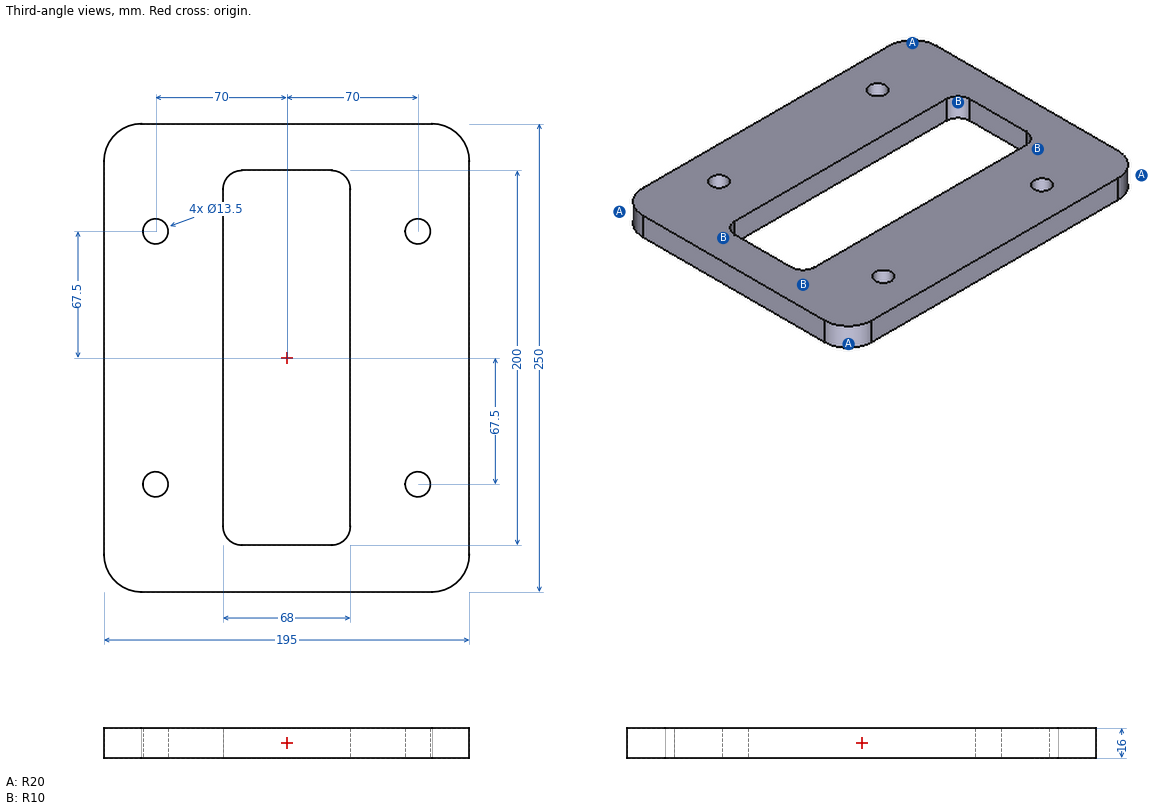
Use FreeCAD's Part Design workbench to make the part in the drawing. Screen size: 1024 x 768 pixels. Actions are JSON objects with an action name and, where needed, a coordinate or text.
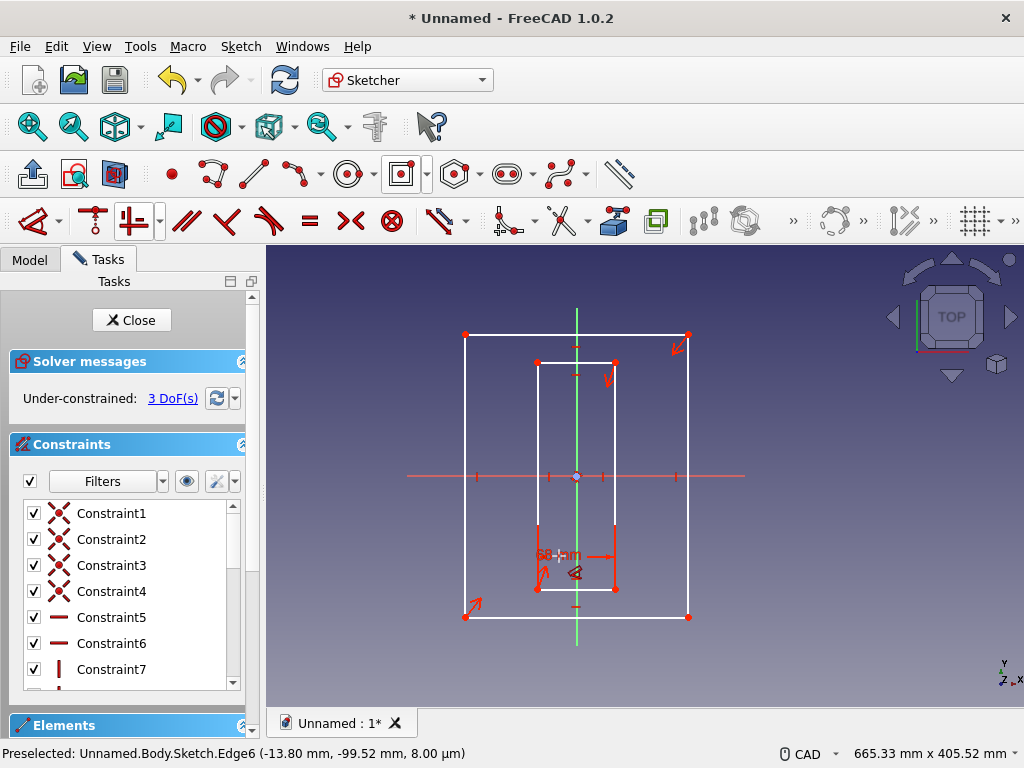
{"action": "left_click", "coordinate": [532, 618]}
{"action": "left_click", "coordinate": [526, 652]}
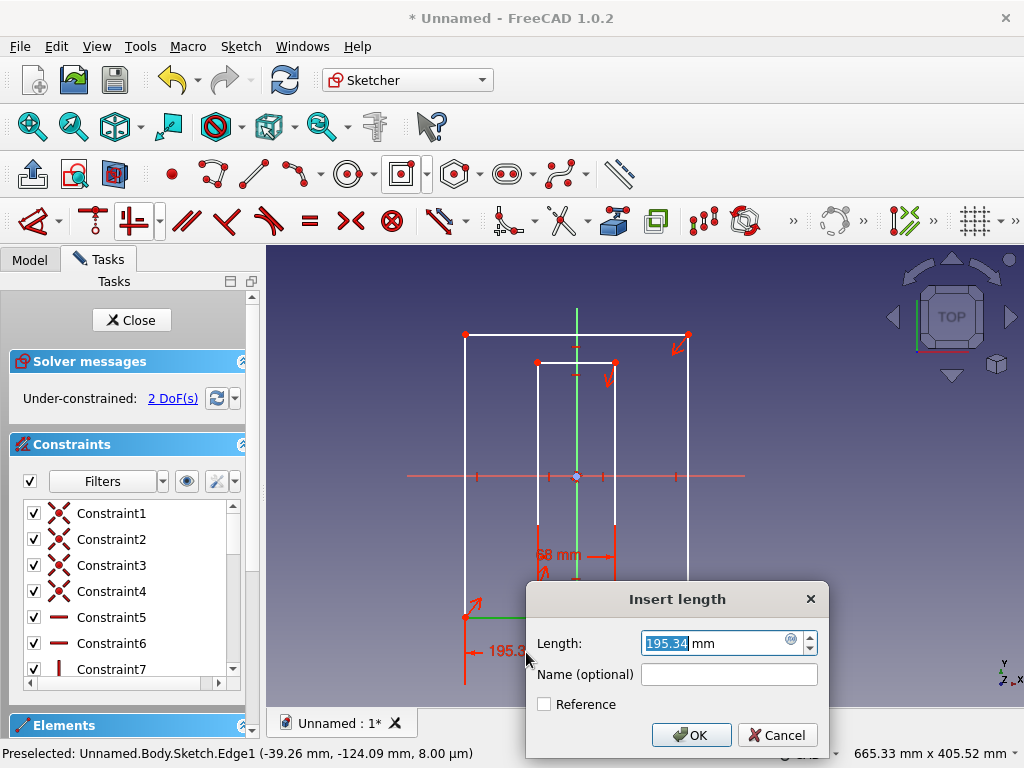
{"action": "type", "text": "195"}
{"action": "key", "text": "Return"}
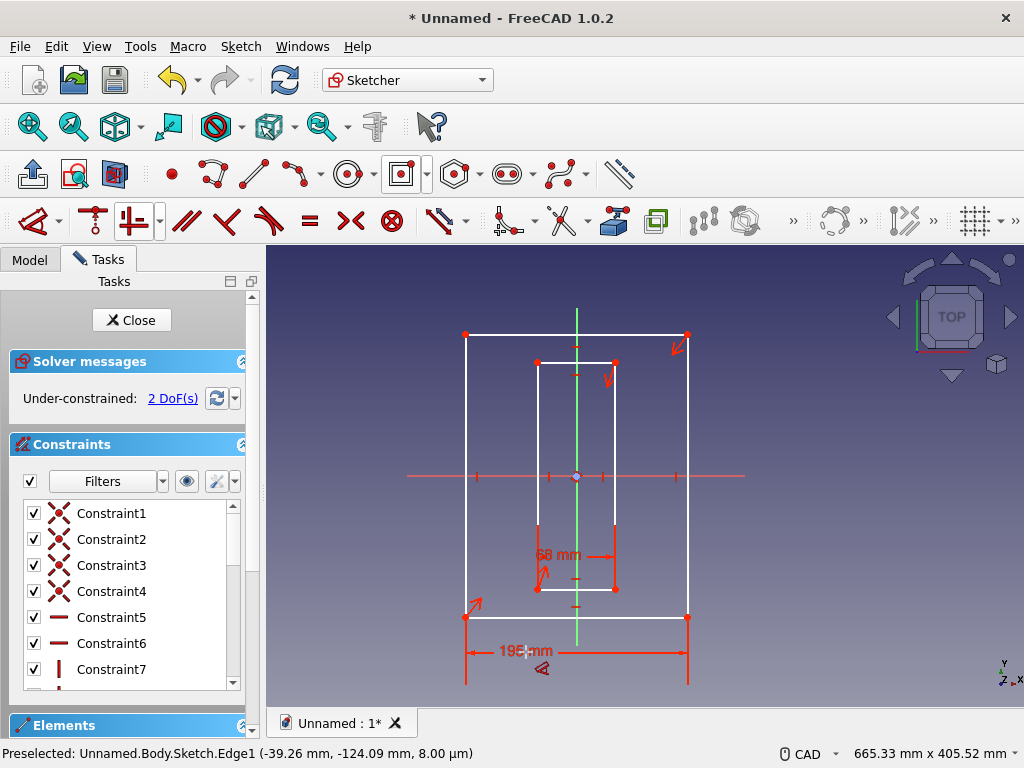
{"action": "left_click", "coordinate": [688, 533]}
{"action": "left_click", "coordinate": [722, 411]}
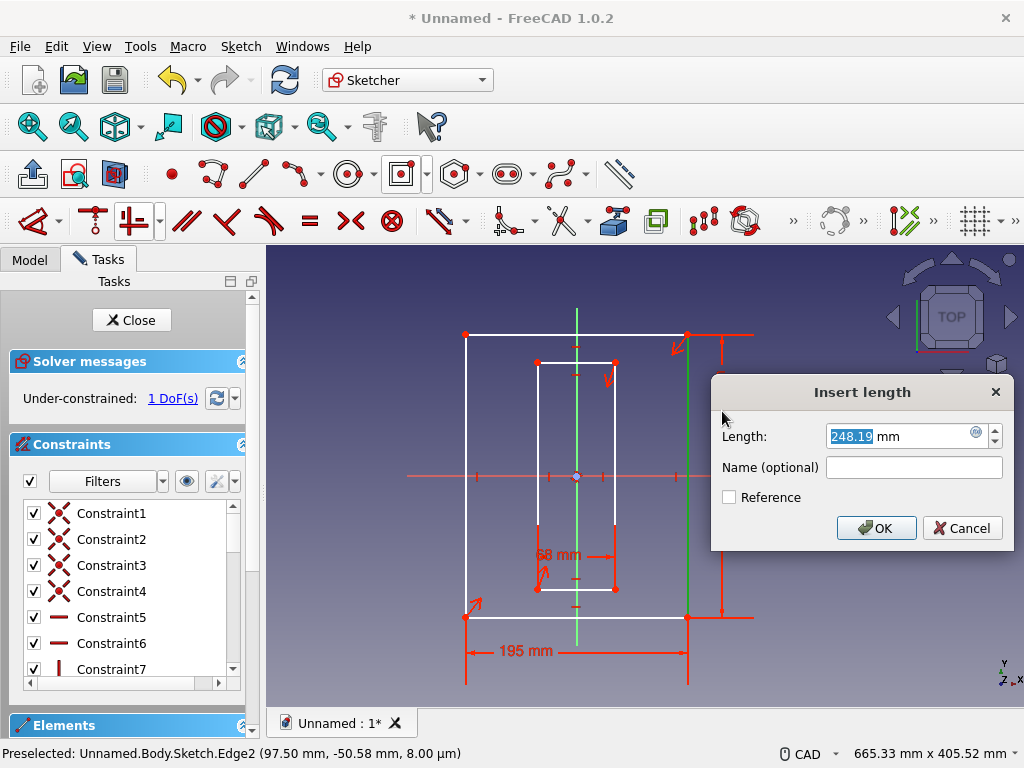
{"action": "type", "text": "250"}
{"action": "key", "text": "Return"}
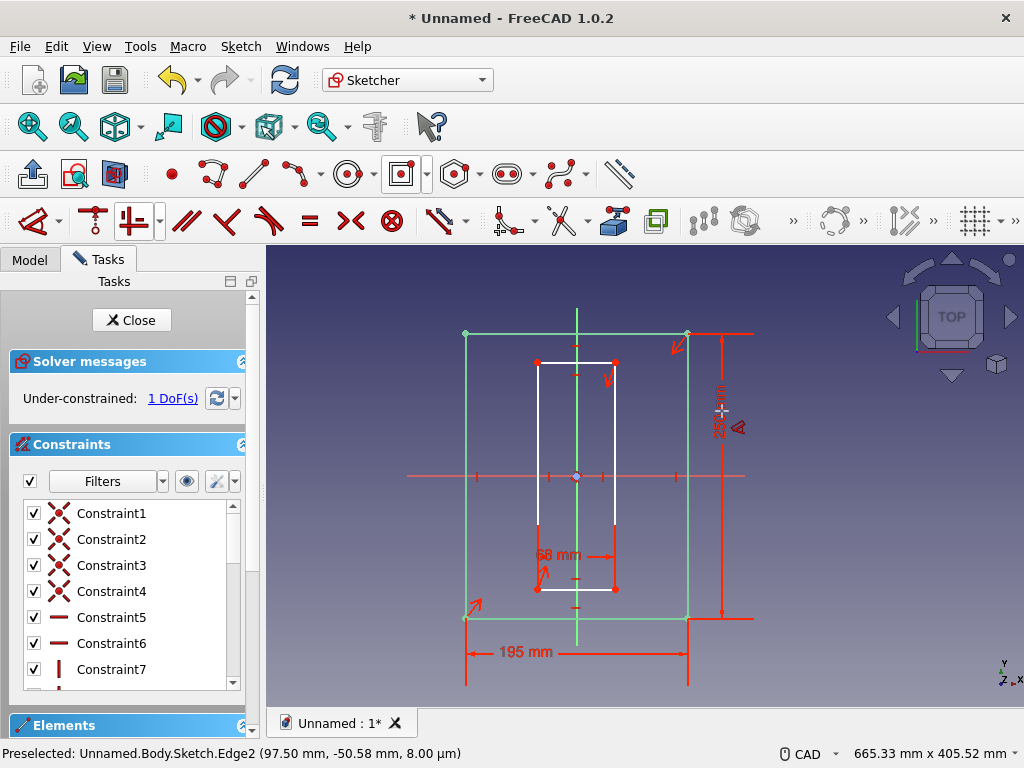
{"action": "left_click", "coordinate": [615, 522]}
{"action": "left_click", "coordinate": [649, 424]}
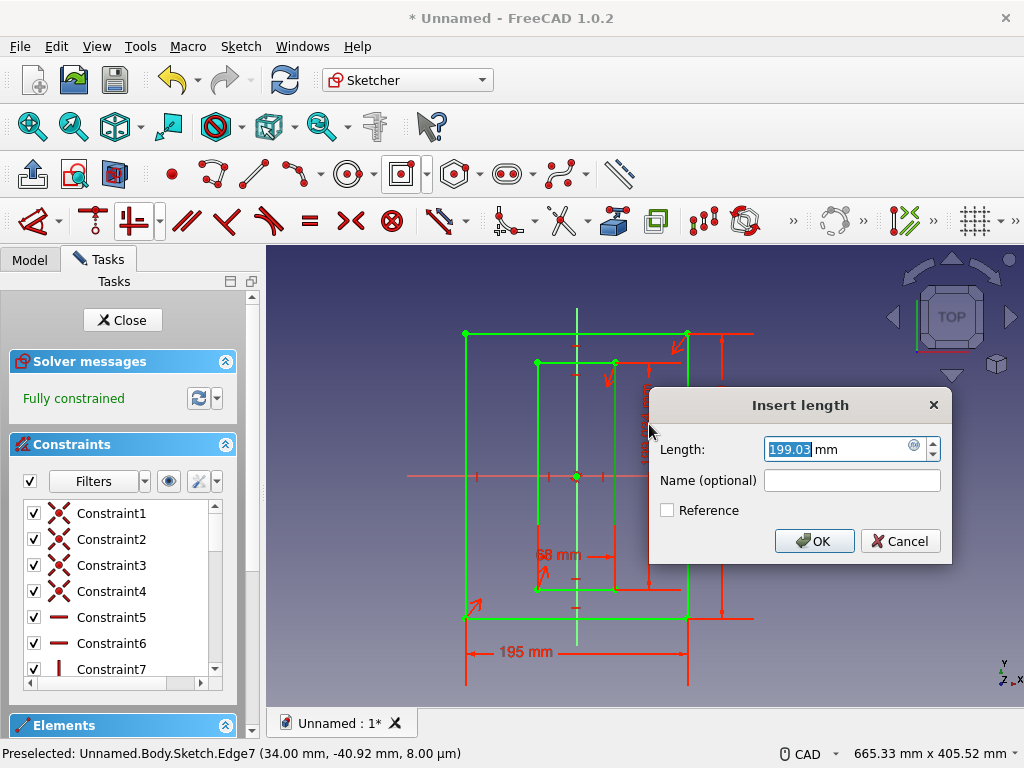
{"action": "type", "text": "200"}
{"action": "key", "text": "Return"}
{"action": "key", "text": "Escape"}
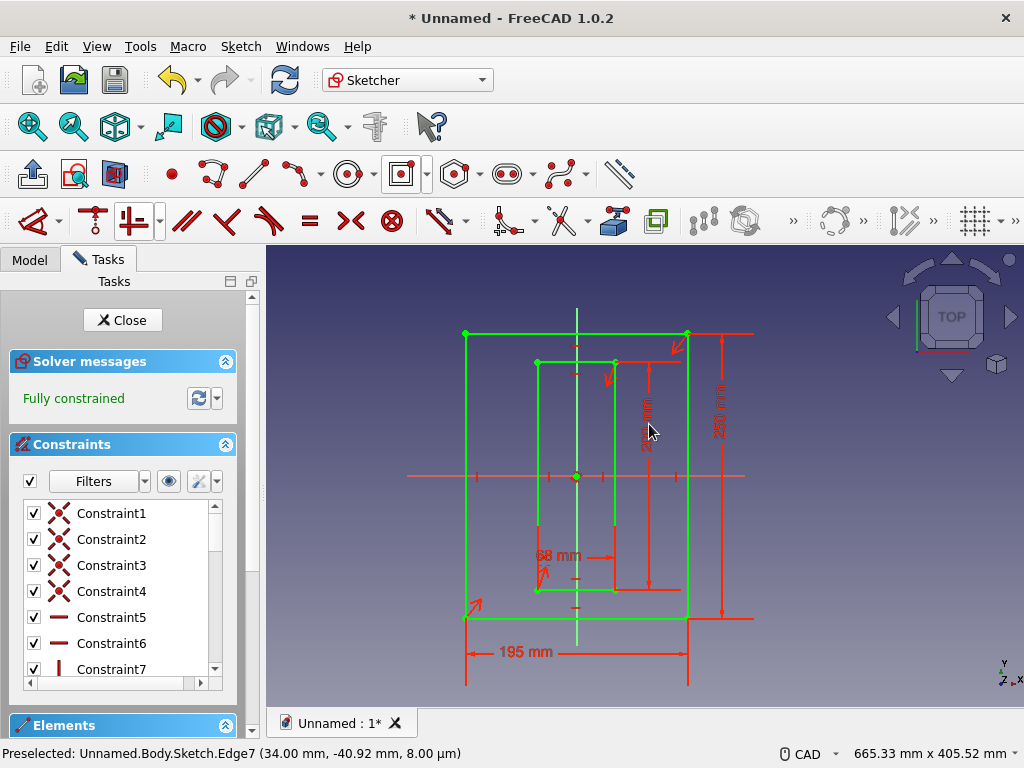
{"action": "left_click", "coordinate": [123, 320]}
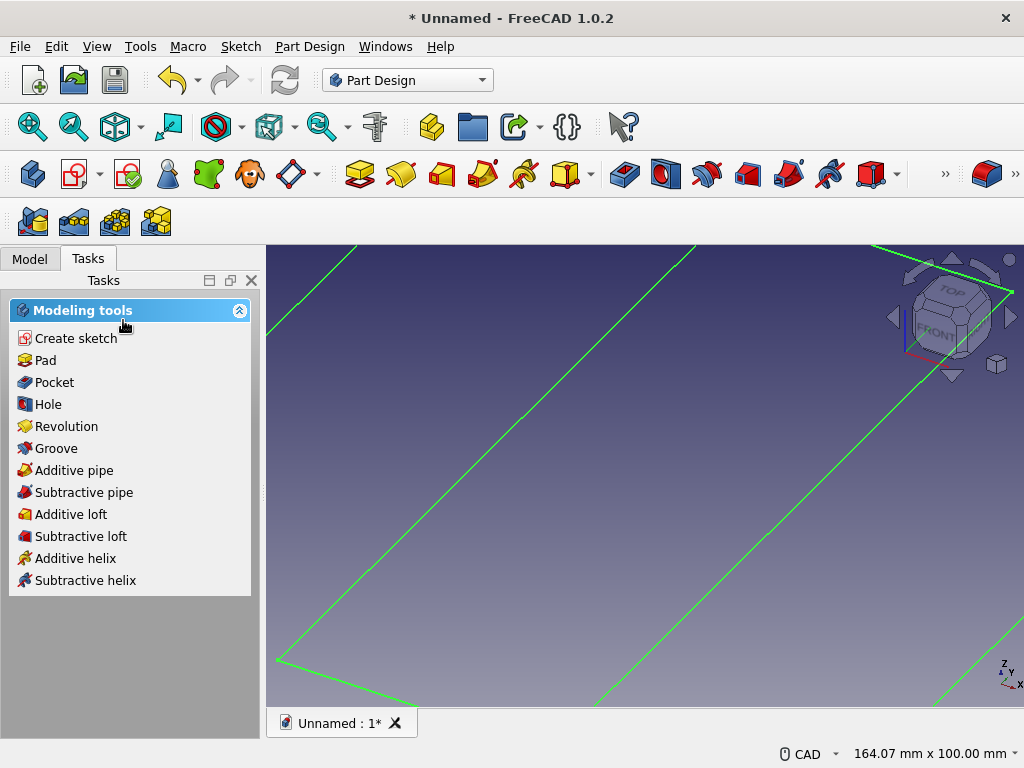
{"action": "left_click", "coordinate": [360, 174]}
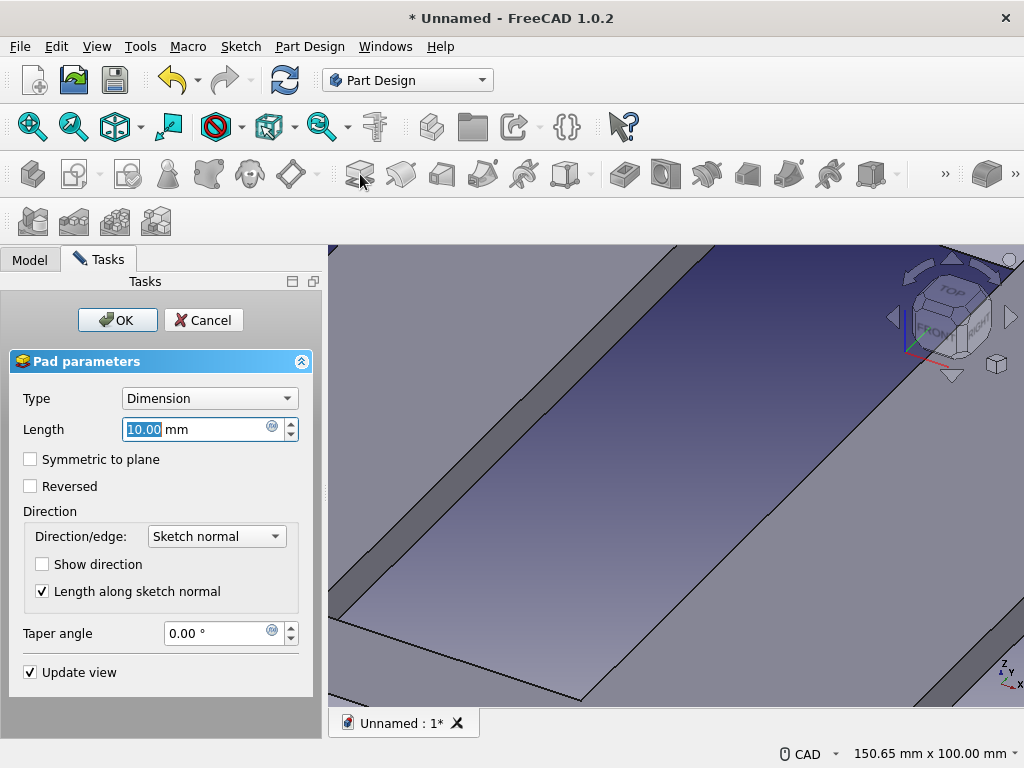
{"action": "type", "text": "16"}
{"action": "key", "text": "Tab"}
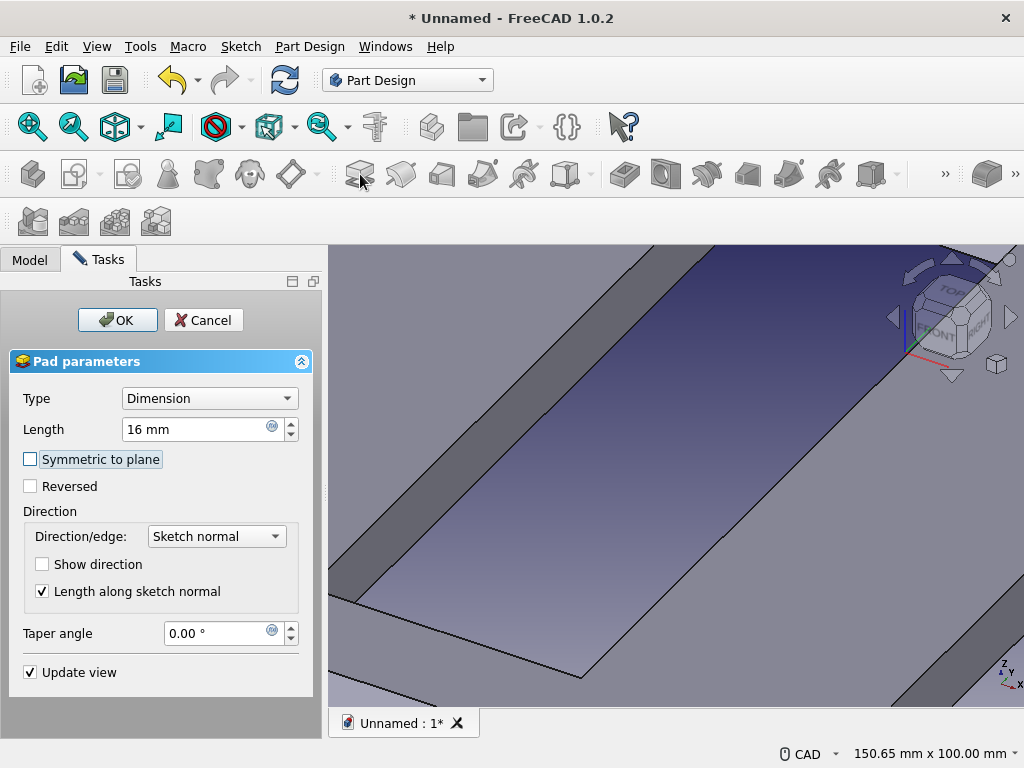
{"action": "left_click", "coordinate": [31, 459]}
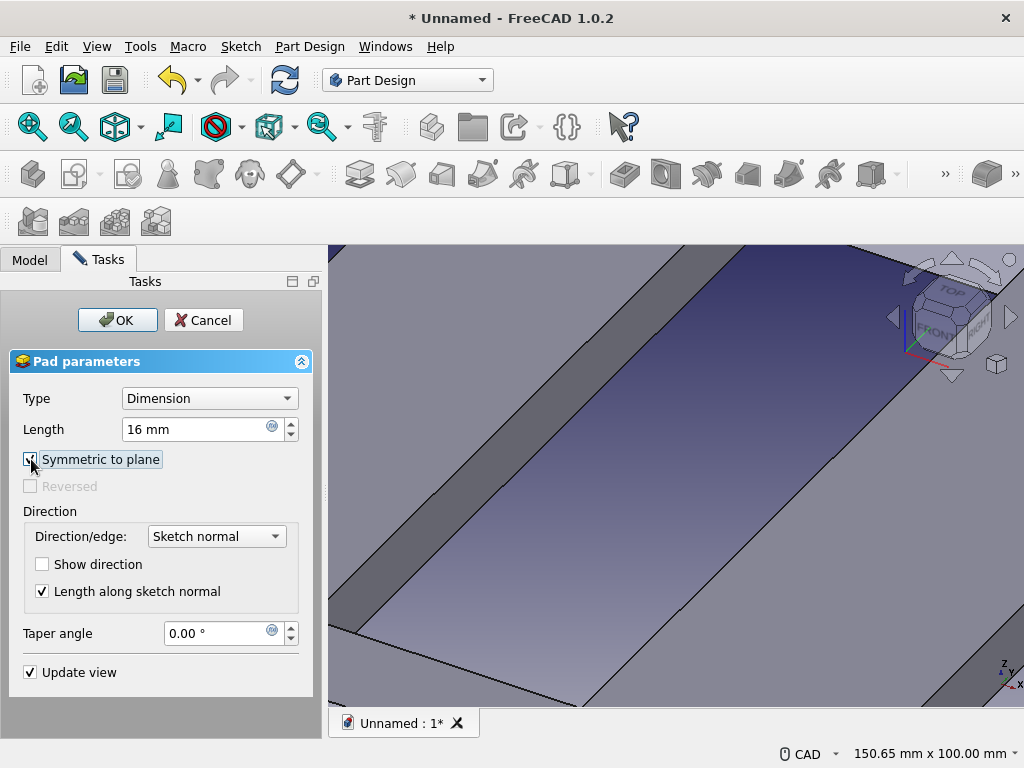
{"action": "left_click", "coordinate": [118, 320]}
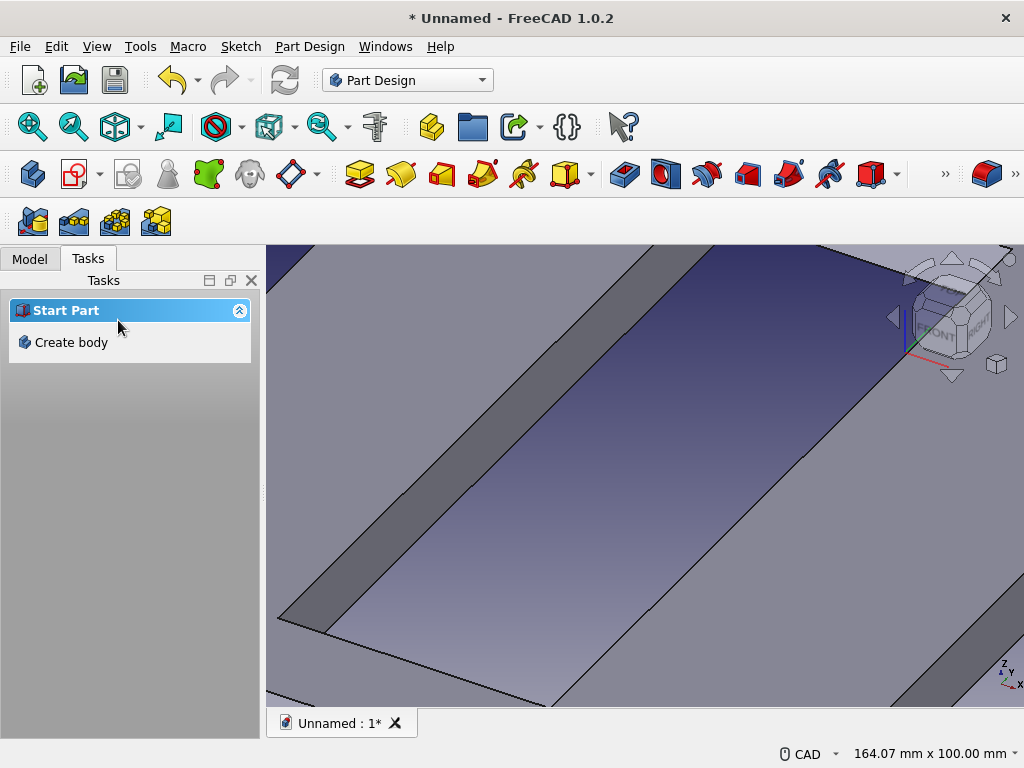
{"action": "left_click", "coordinate": [33, 128]}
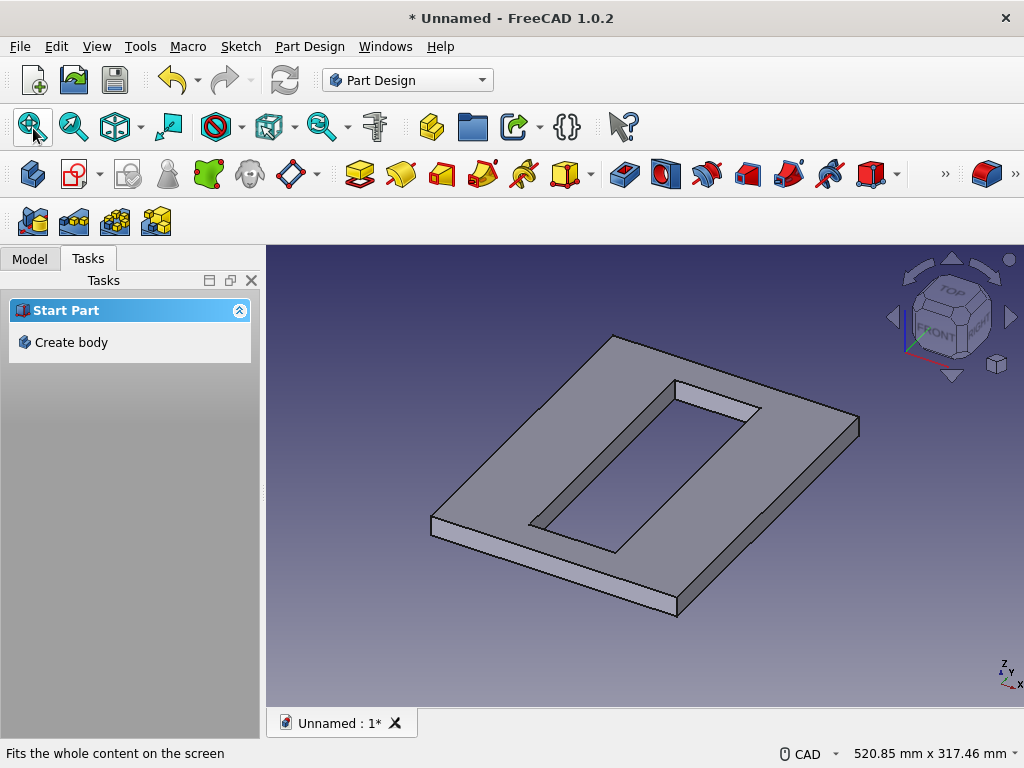
{"action": "left_click", "coordinate": [767, 437]}